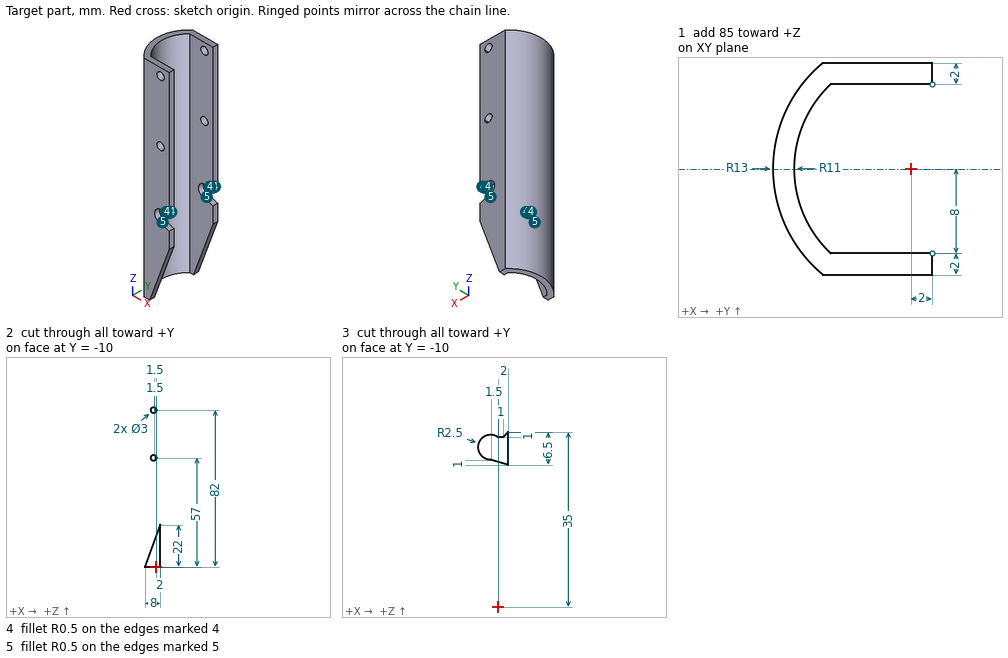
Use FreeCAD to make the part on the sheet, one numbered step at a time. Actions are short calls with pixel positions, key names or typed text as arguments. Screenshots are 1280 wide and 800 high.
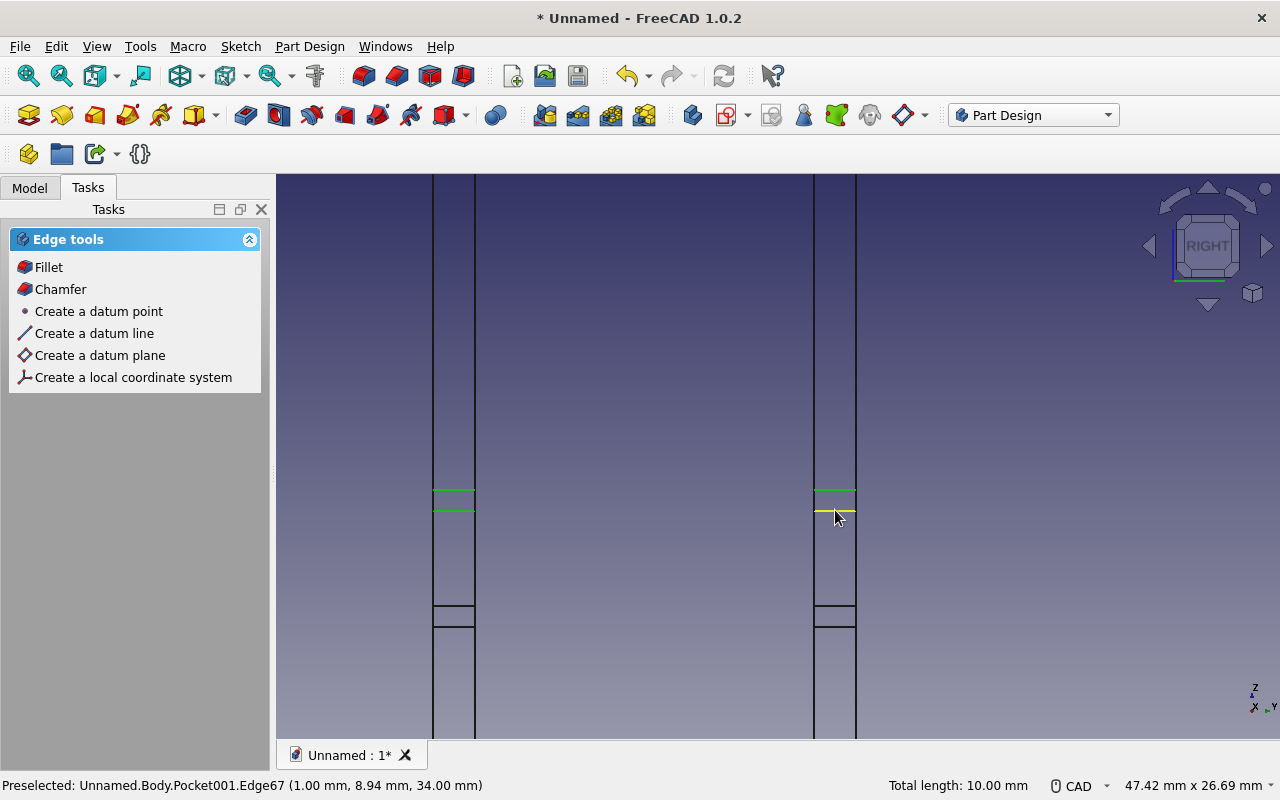
click(835, 510, ctrl)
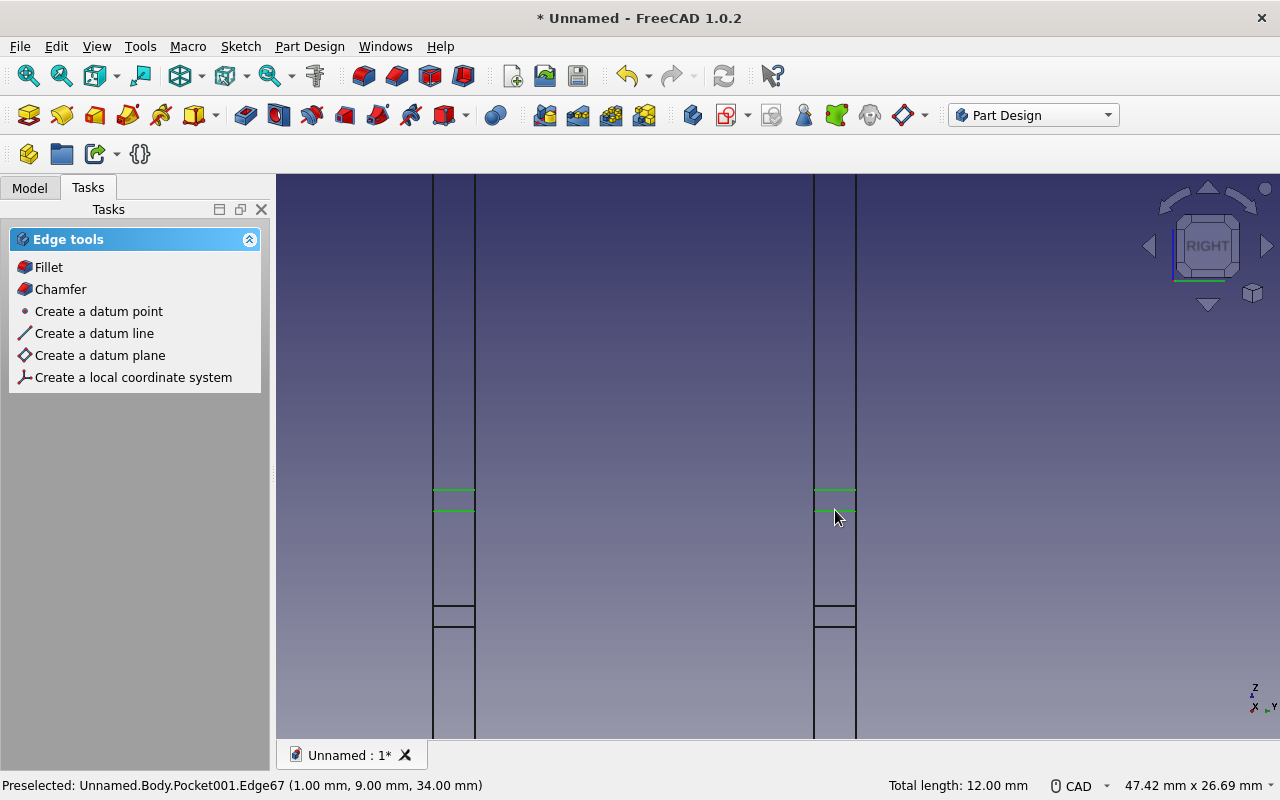
key(v)
key(1)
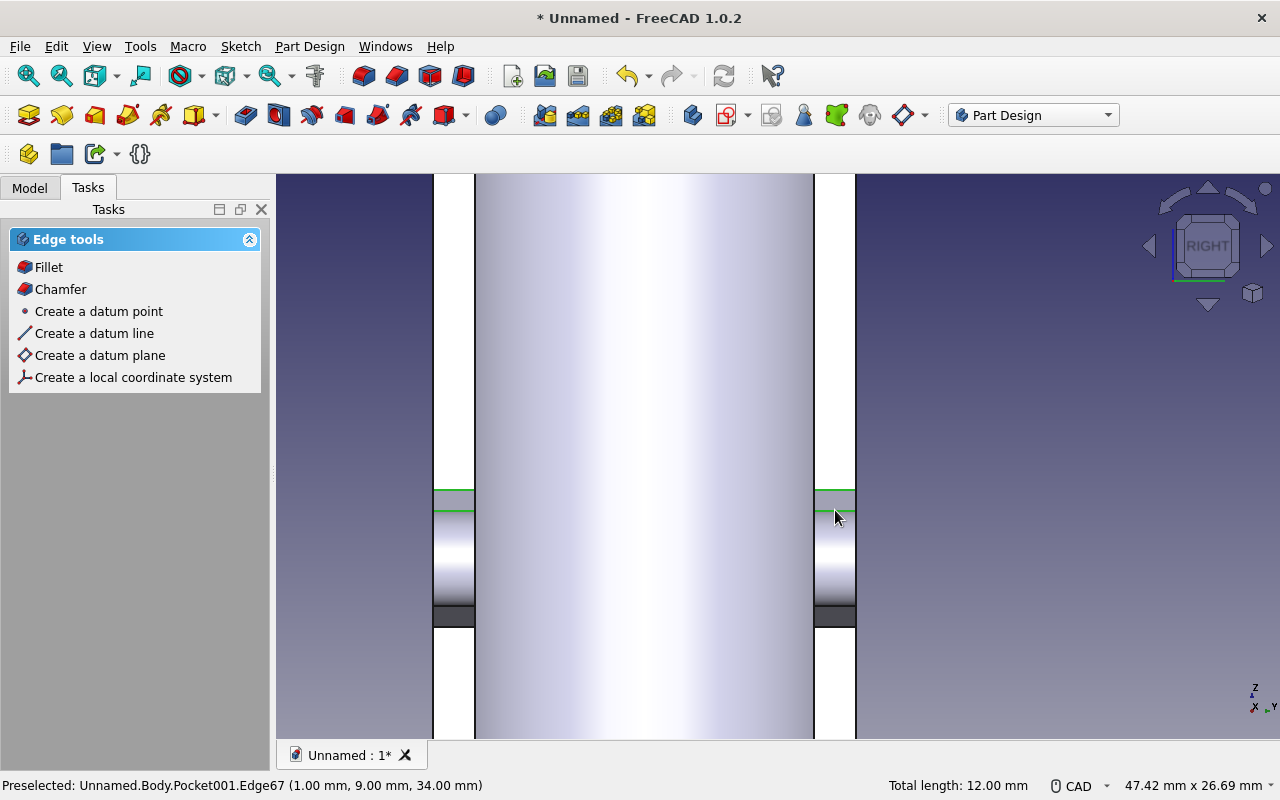
click(364, 76)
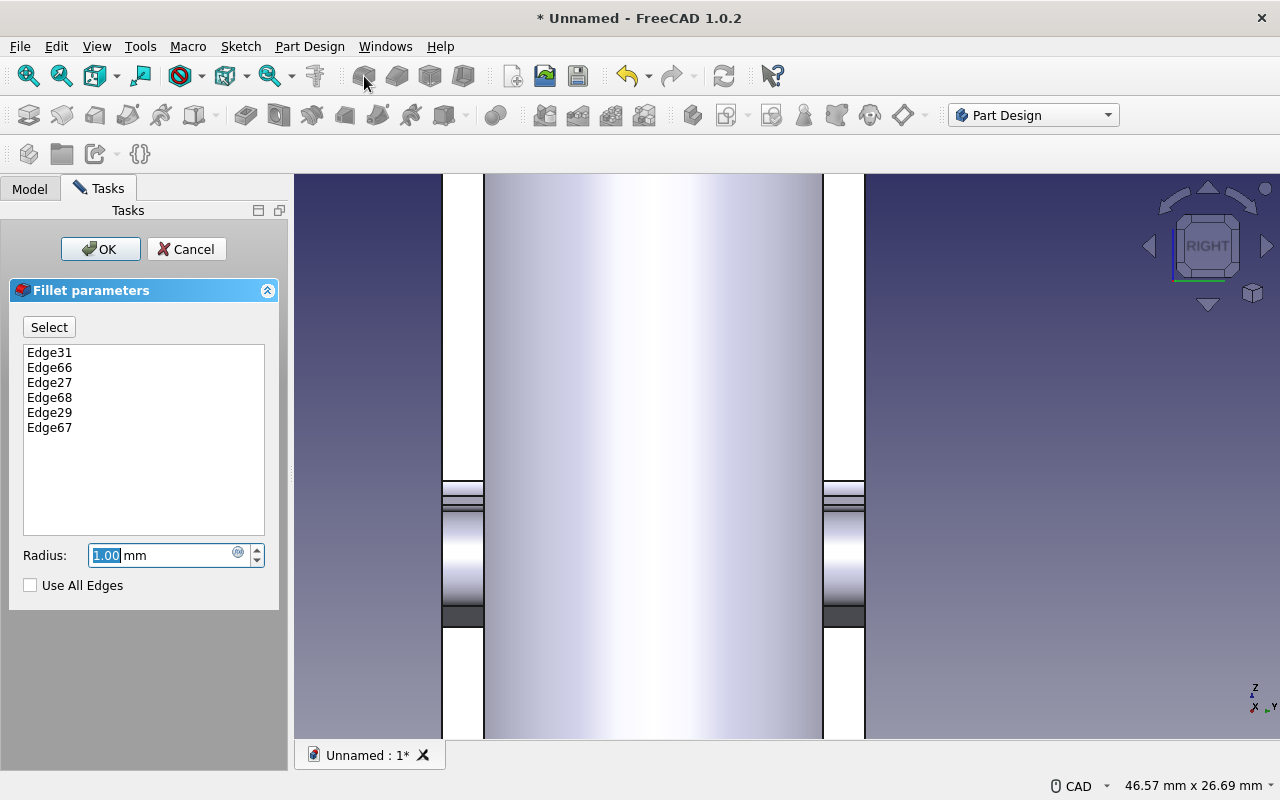
text(0.5)
key(Tab)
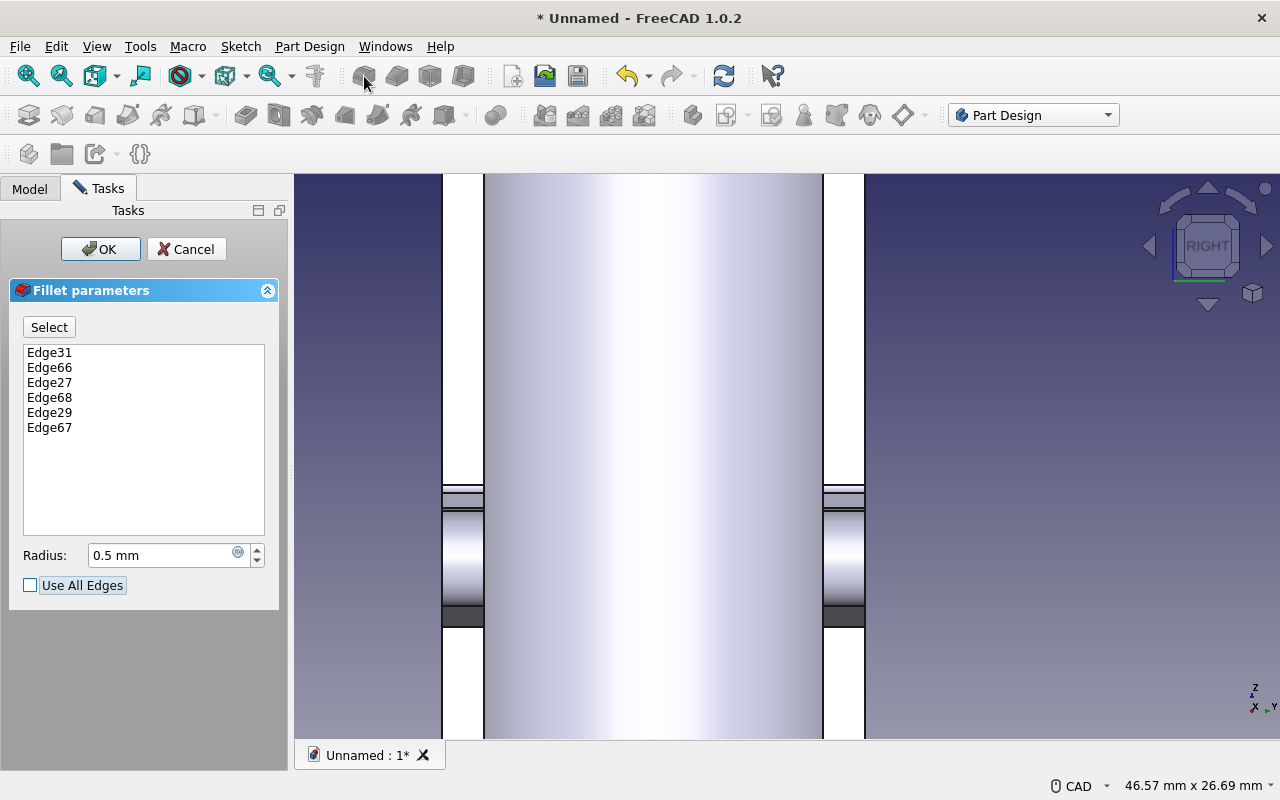
click(101, 249)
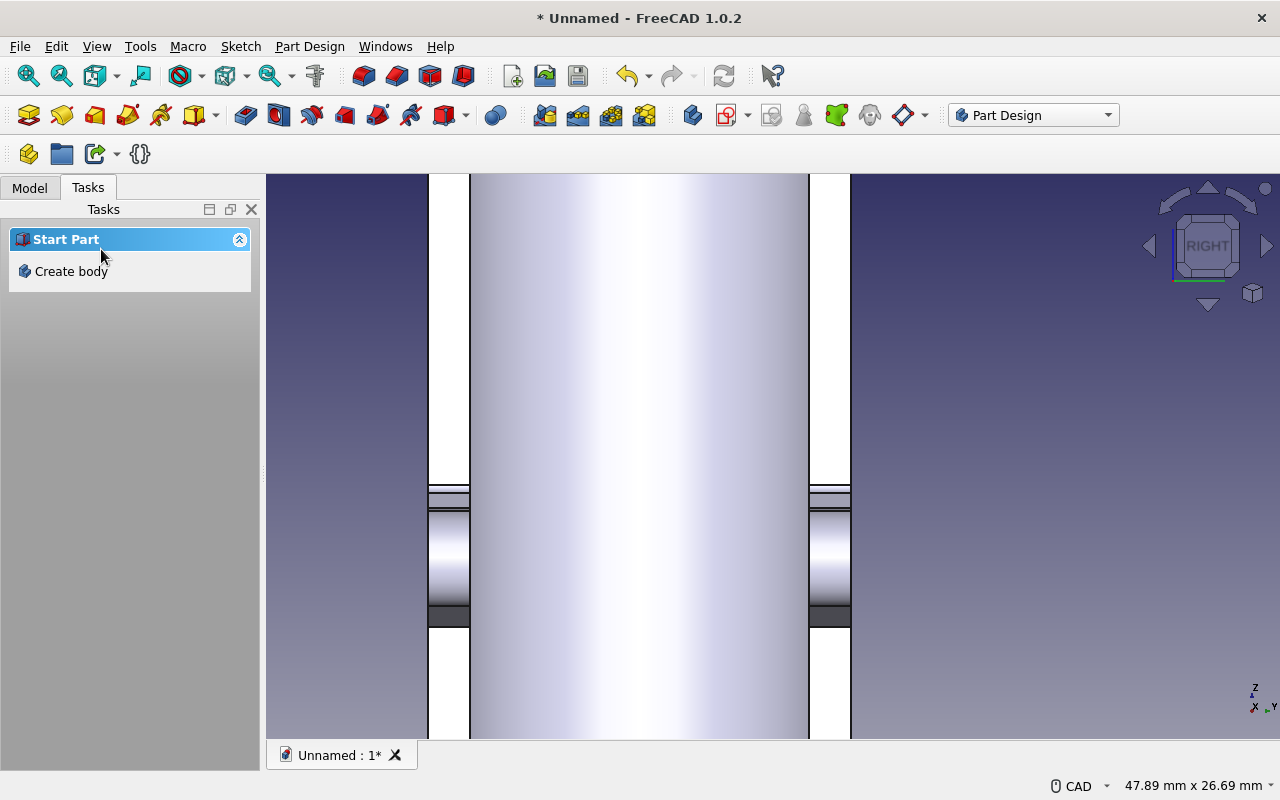
click(29, 76)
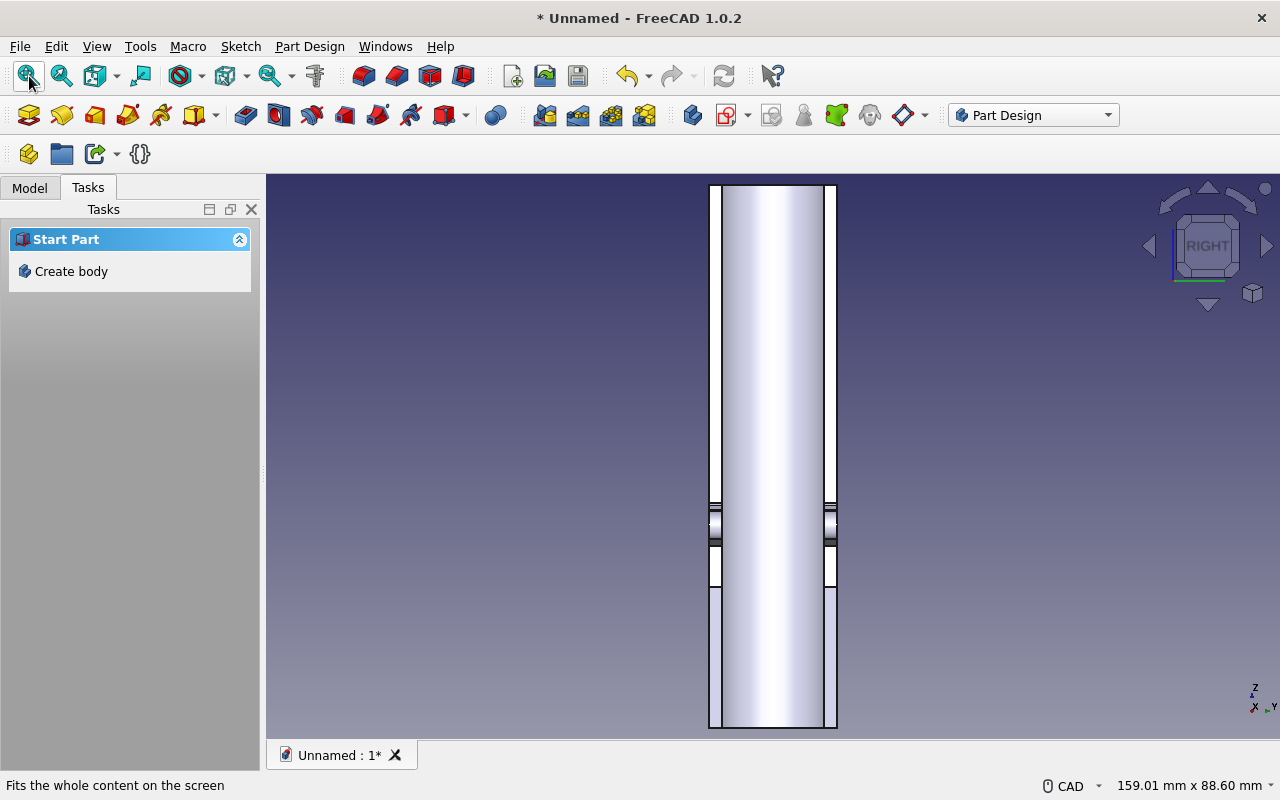
scroll(716, 538, up, 6)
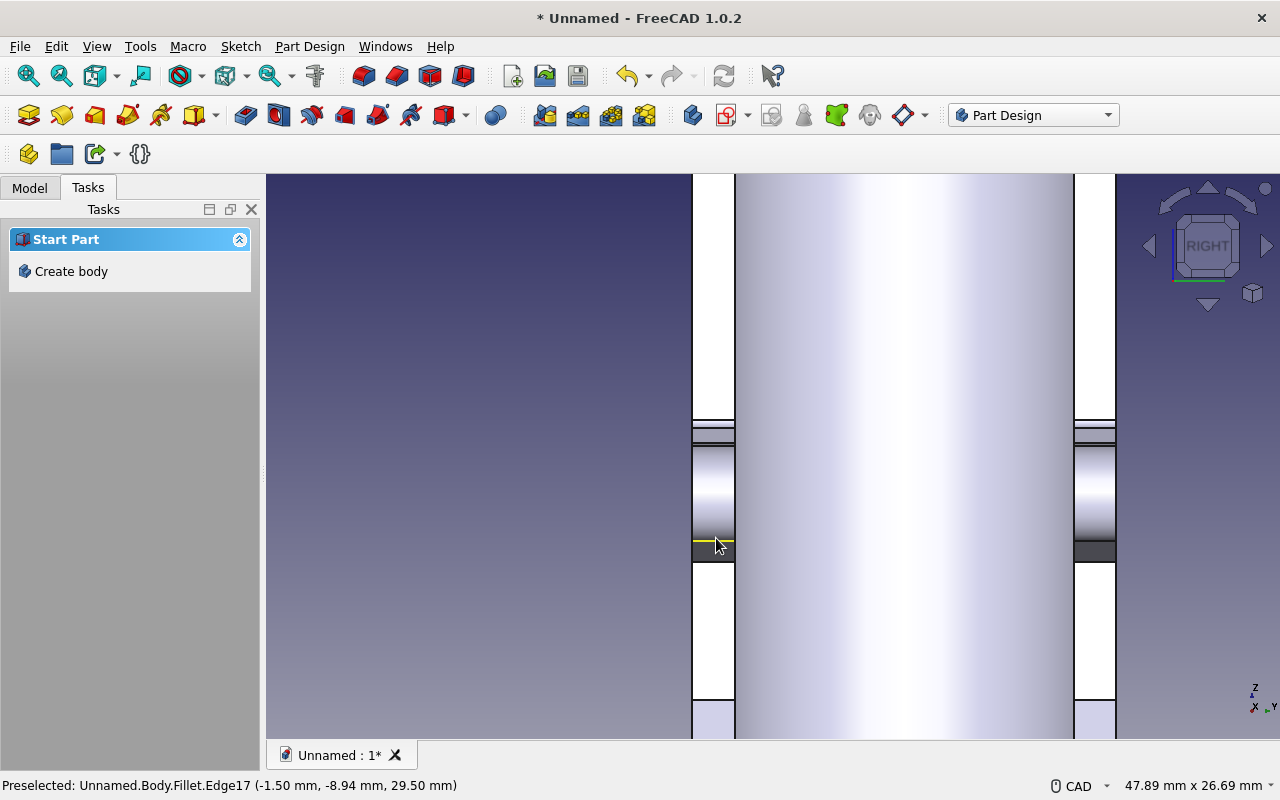
key(v)
key(f)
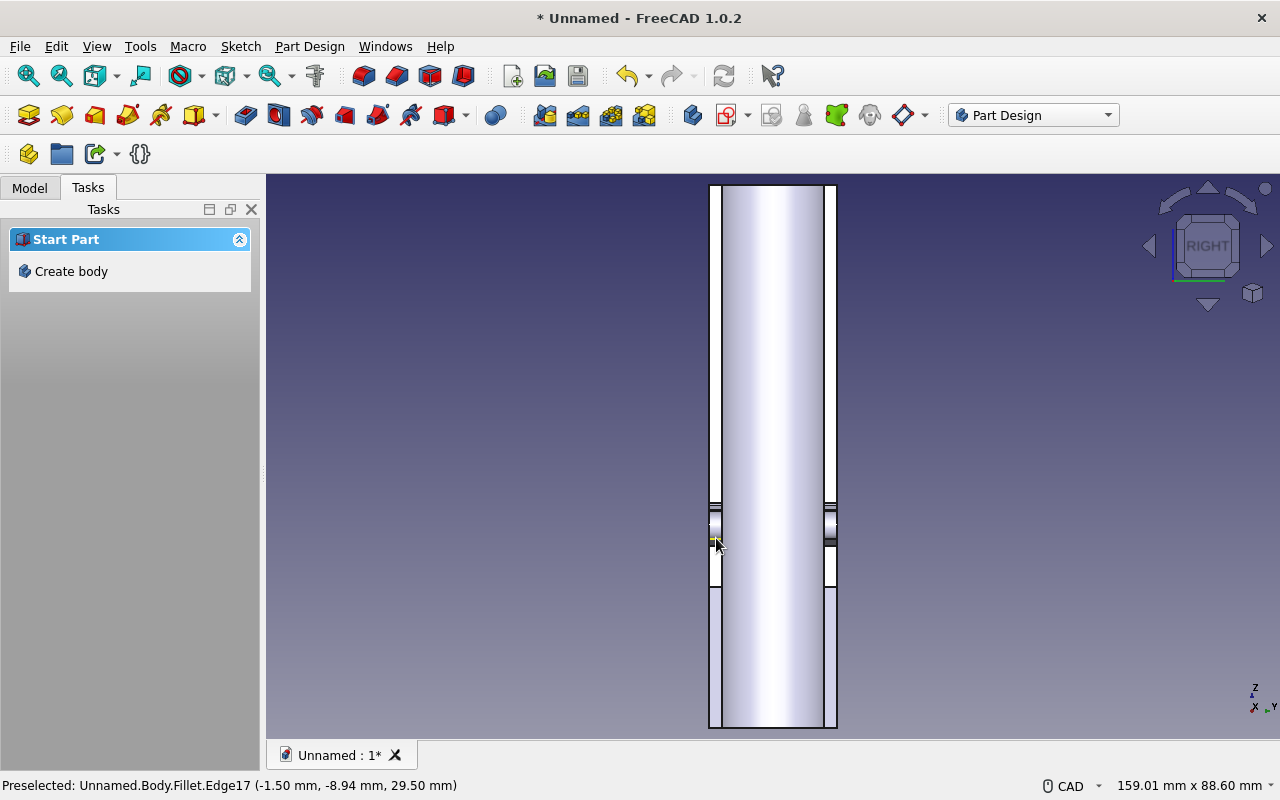
key(0)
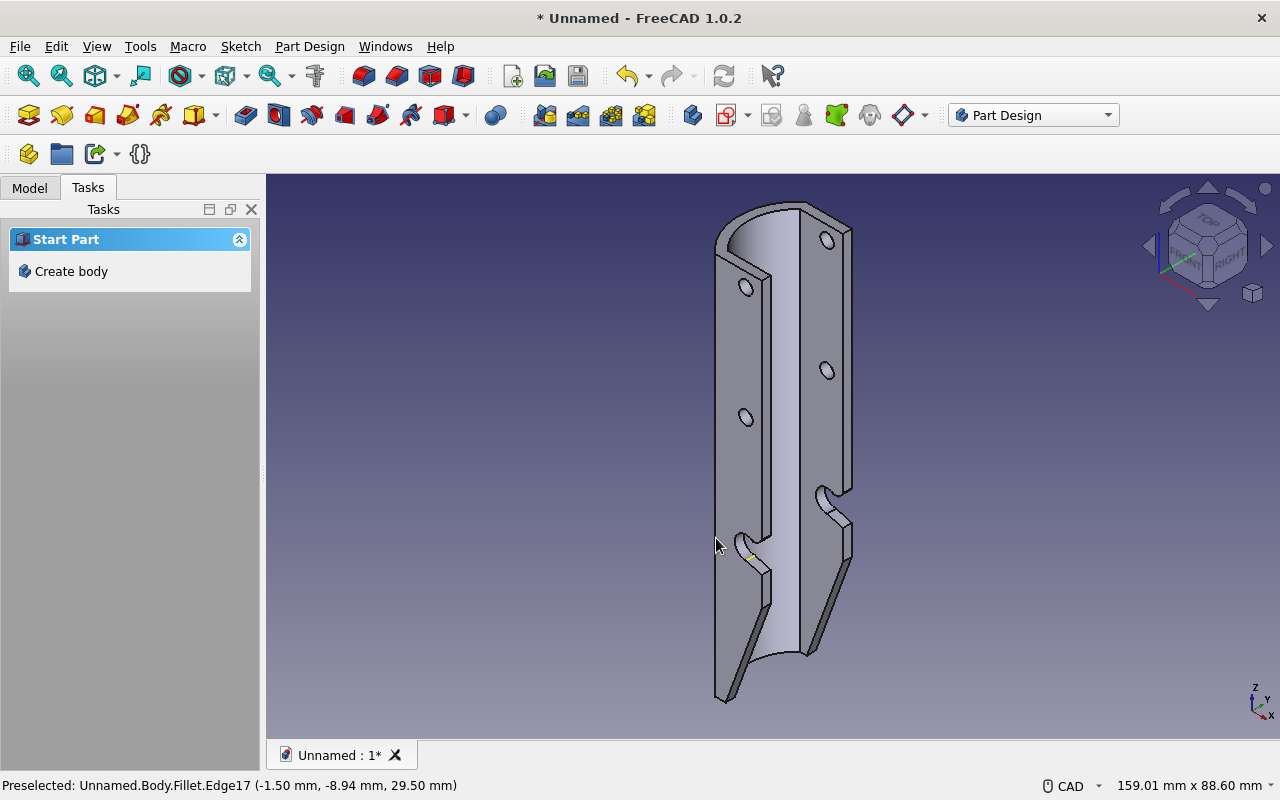
scroll(750, 557, up, 6)